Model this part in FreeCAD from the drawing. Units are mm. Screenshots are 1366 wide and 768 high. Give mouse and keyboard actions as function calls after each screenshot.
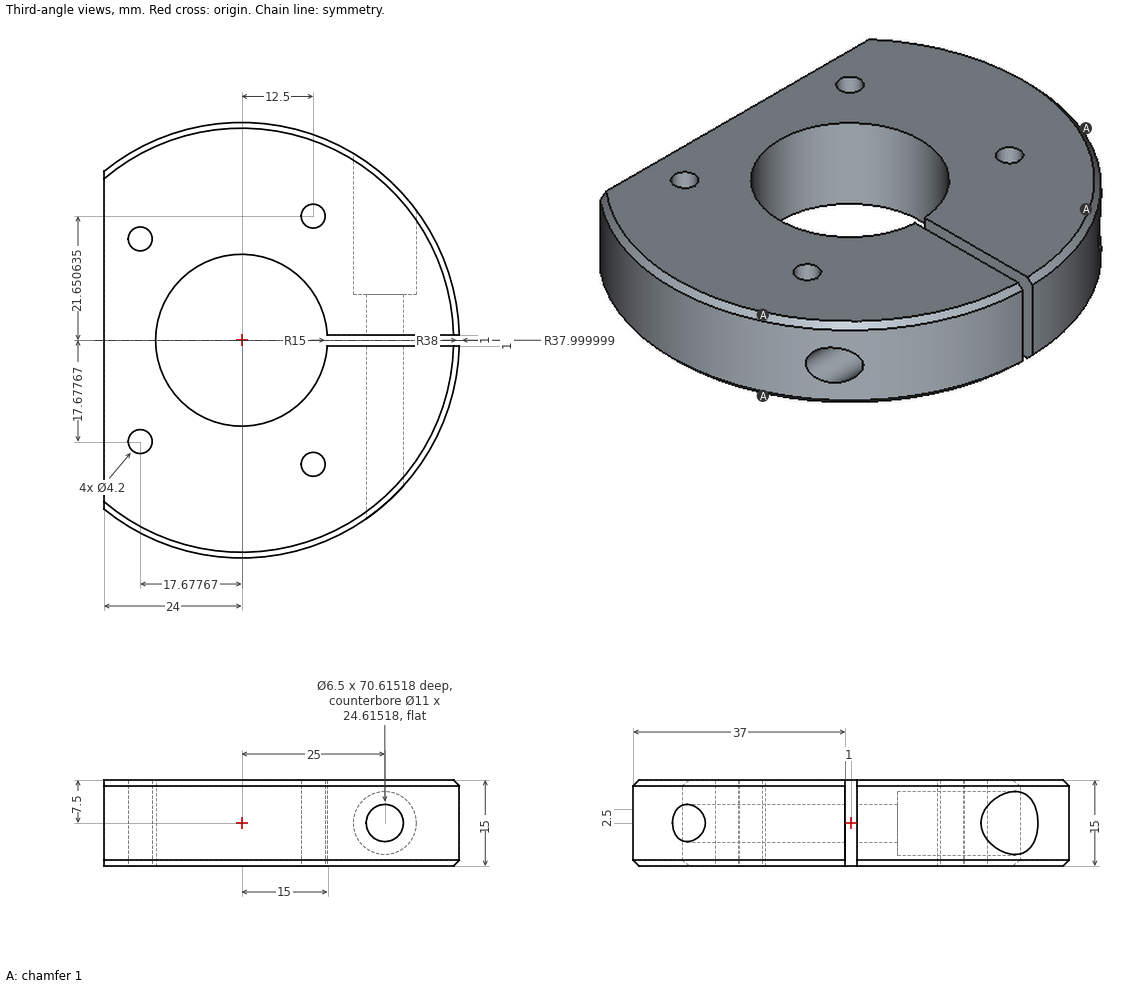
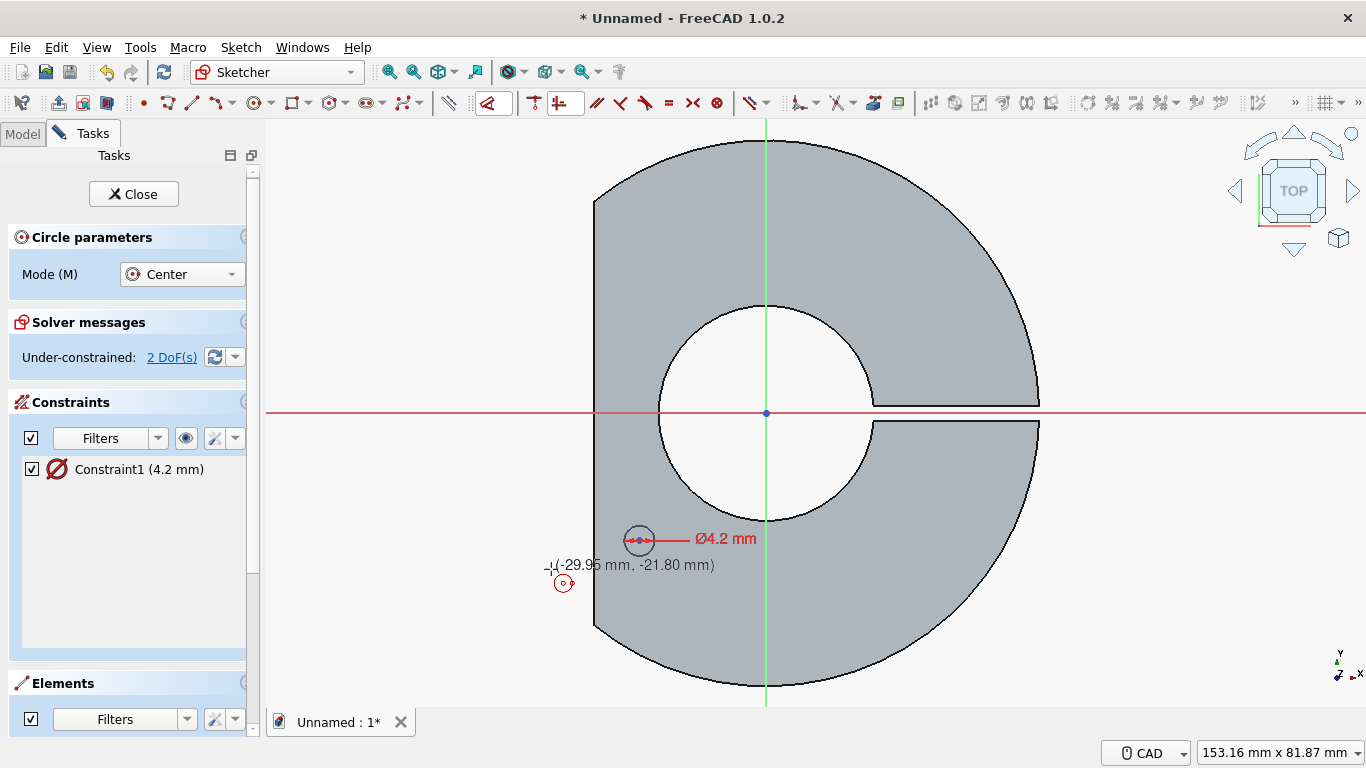
scroll(639, 286, up, 3)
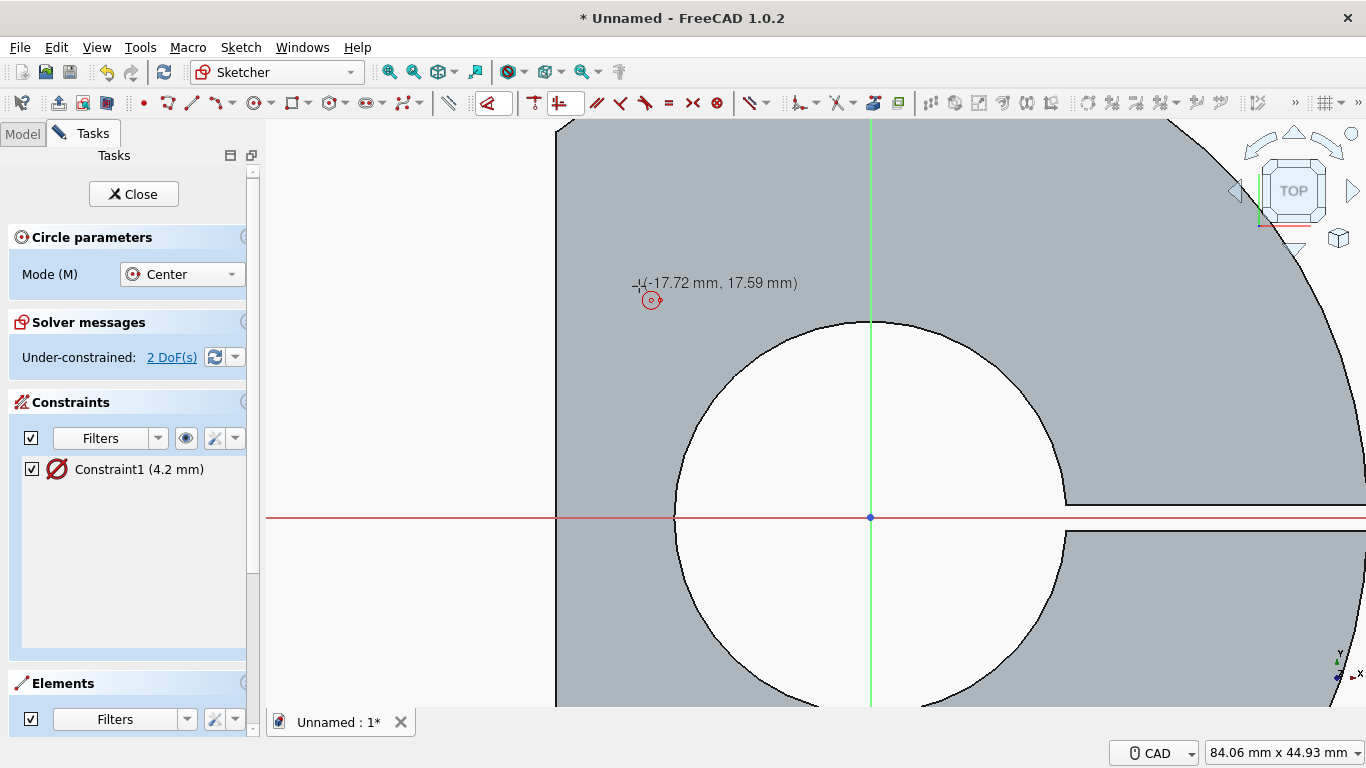
click(639, 286)
move(659, 267)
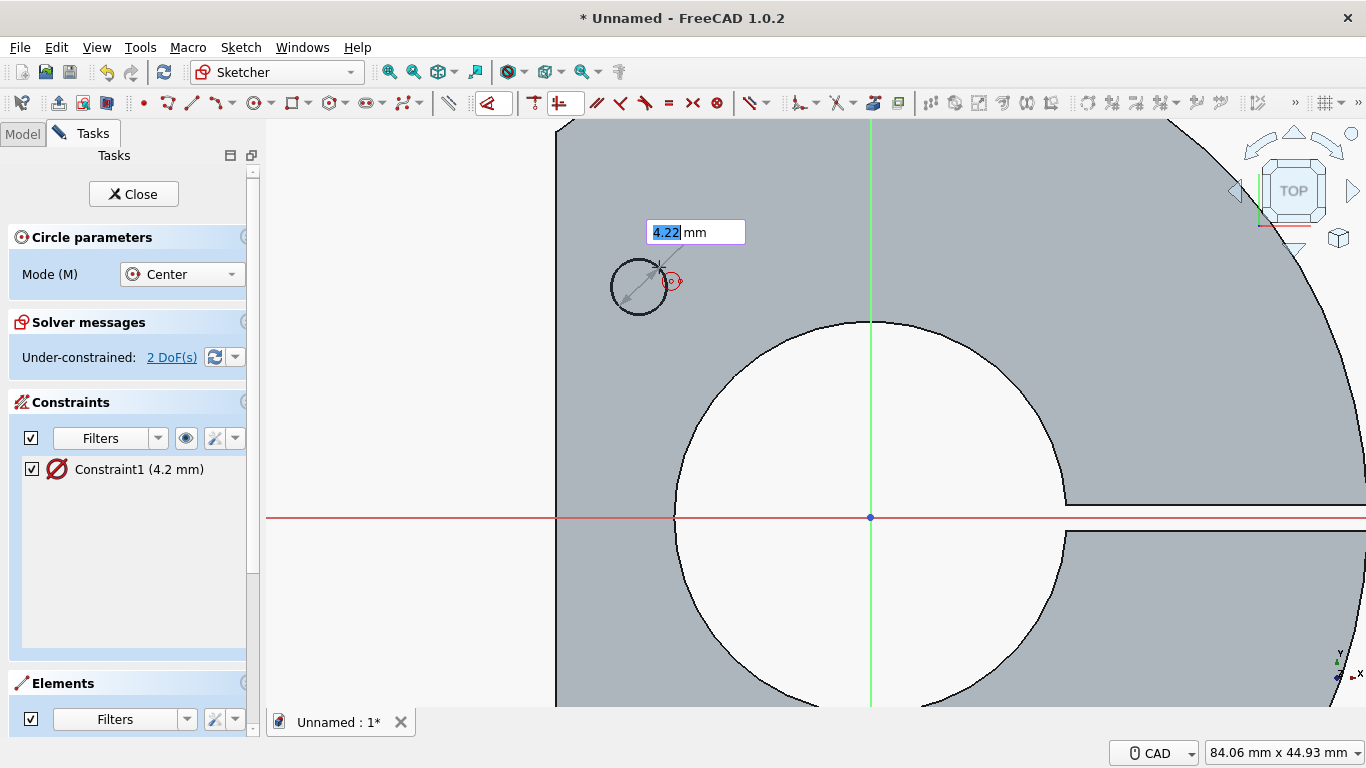
text(4.2)
key(Return)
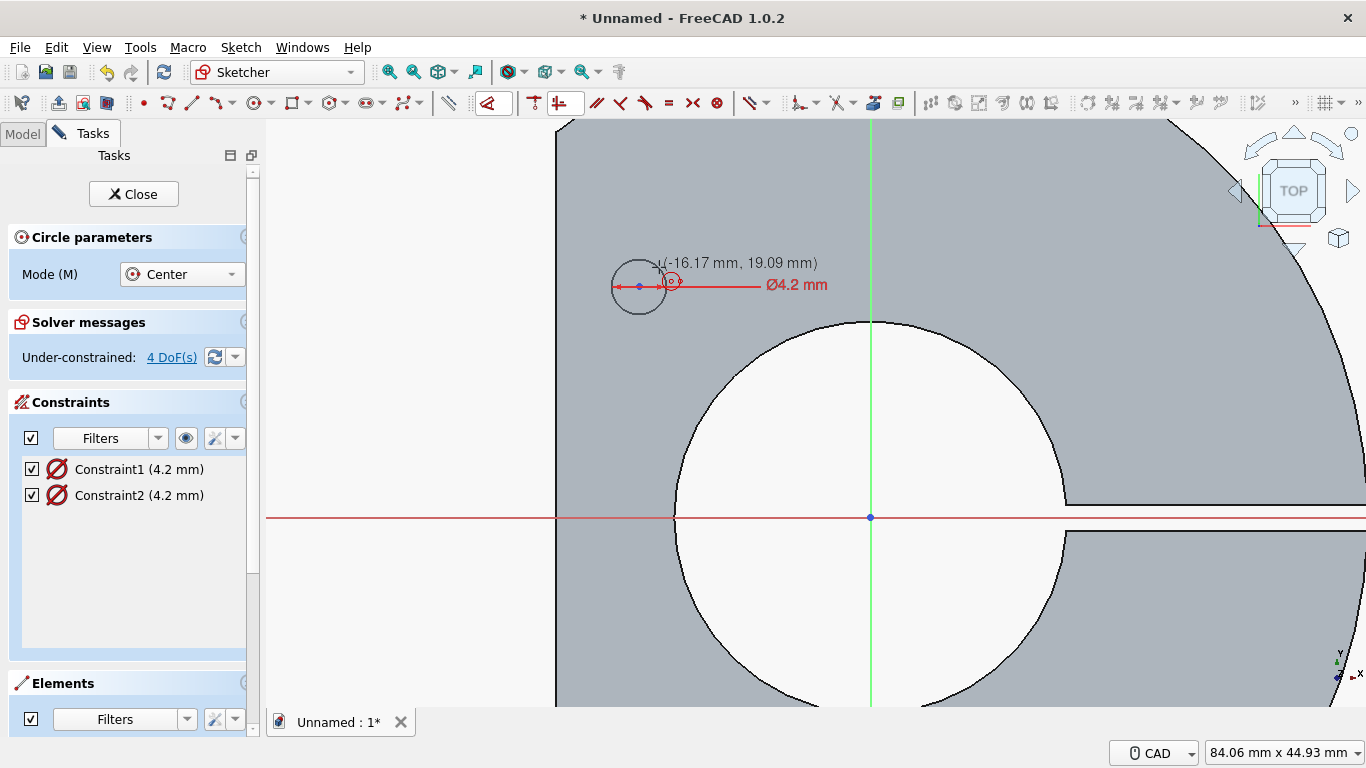
click(1034, 234)
move(1054, 215)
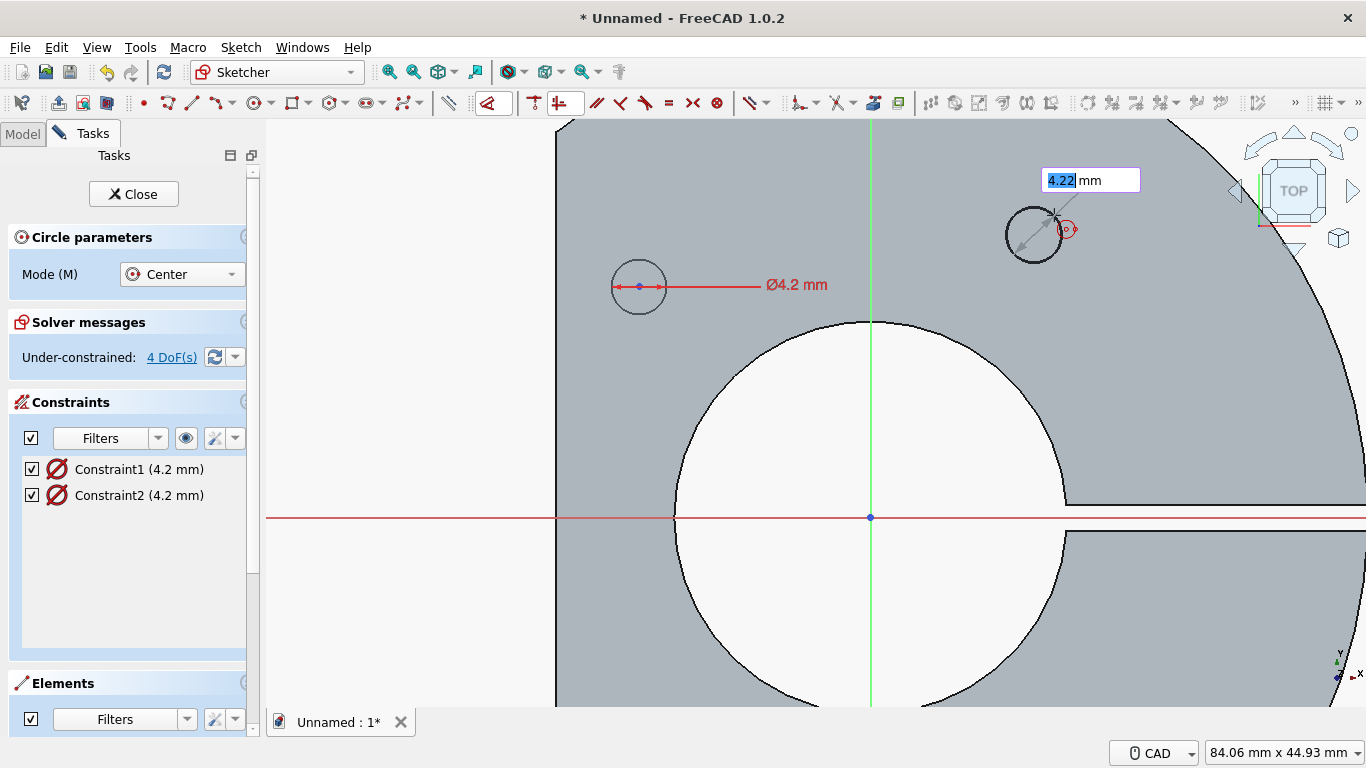
text(4.2)
key(Return)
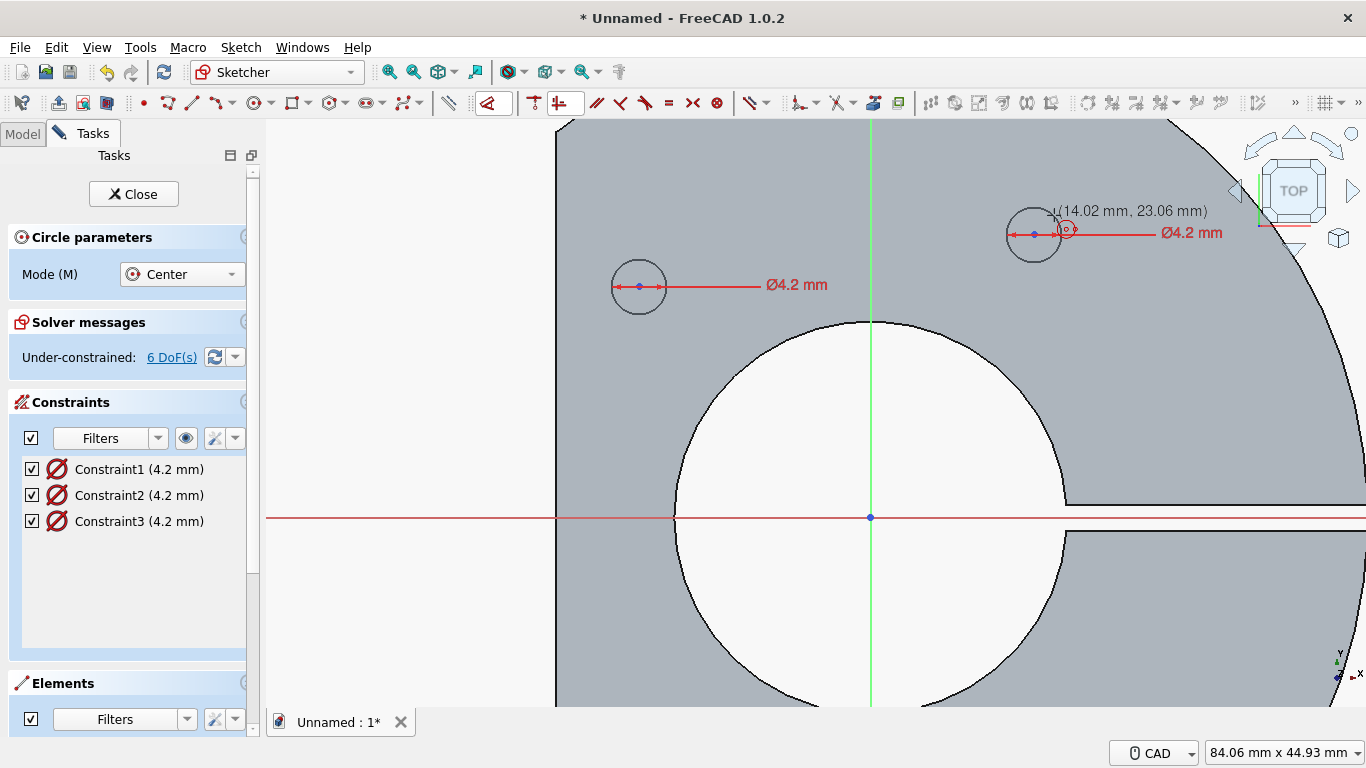
scroll(639, 286, down, 3)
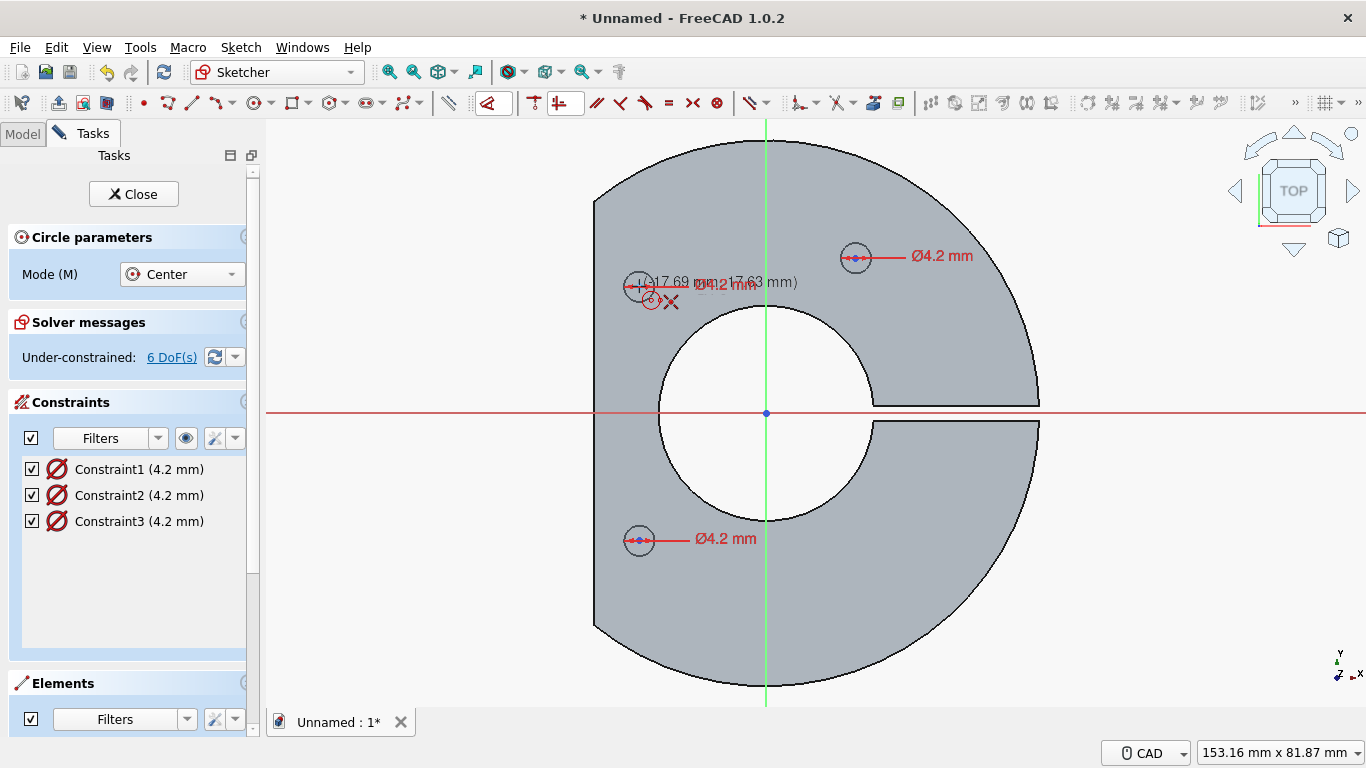
scroll(856, 569, up, 3)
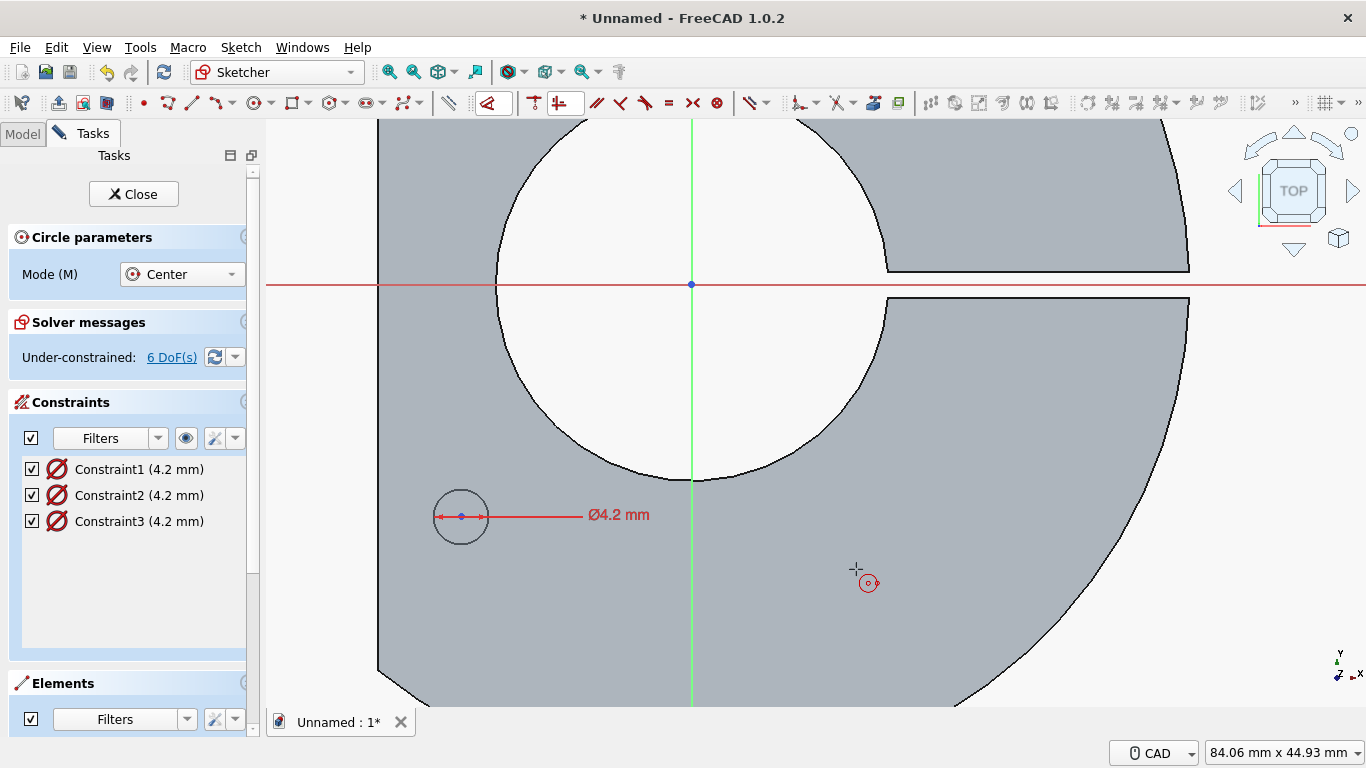
click(856, 568)
move(875, 549)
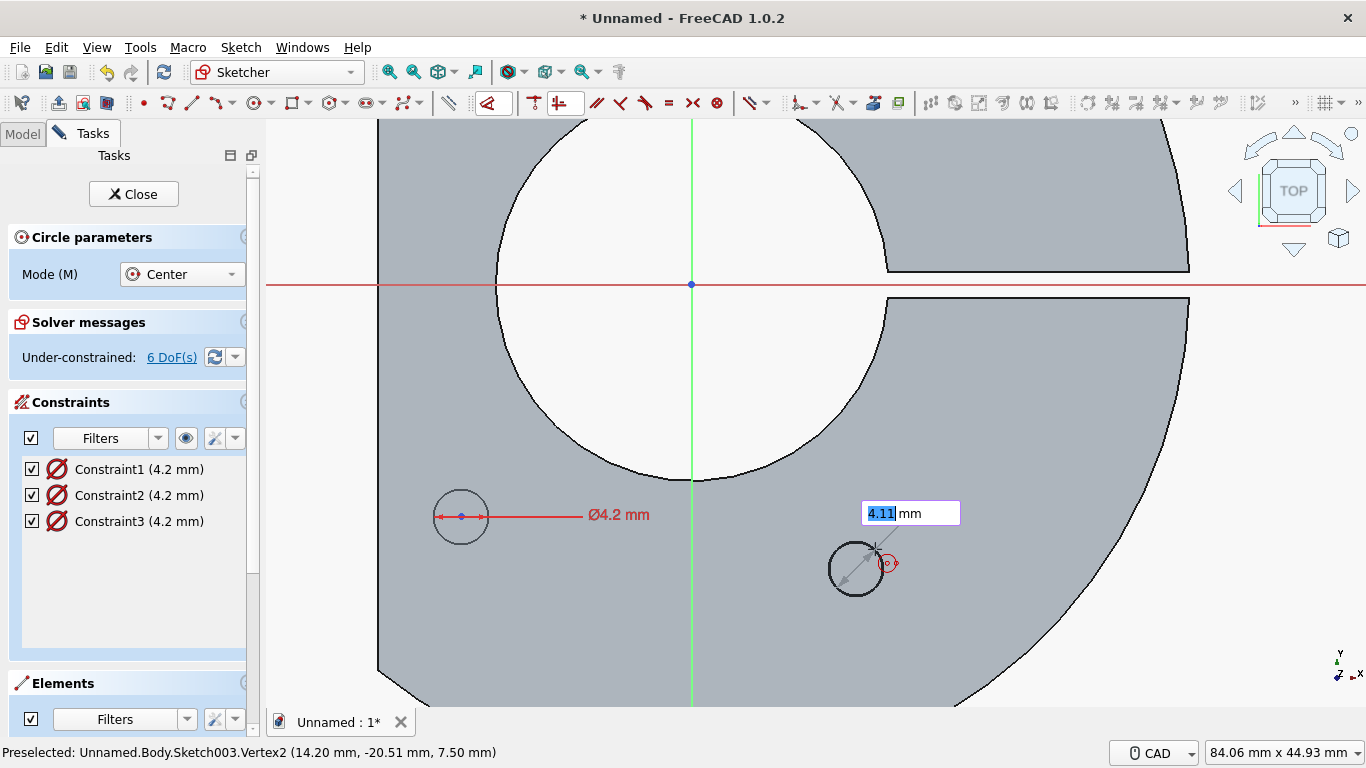
text(4.2)
key(Return)
key(Escape)